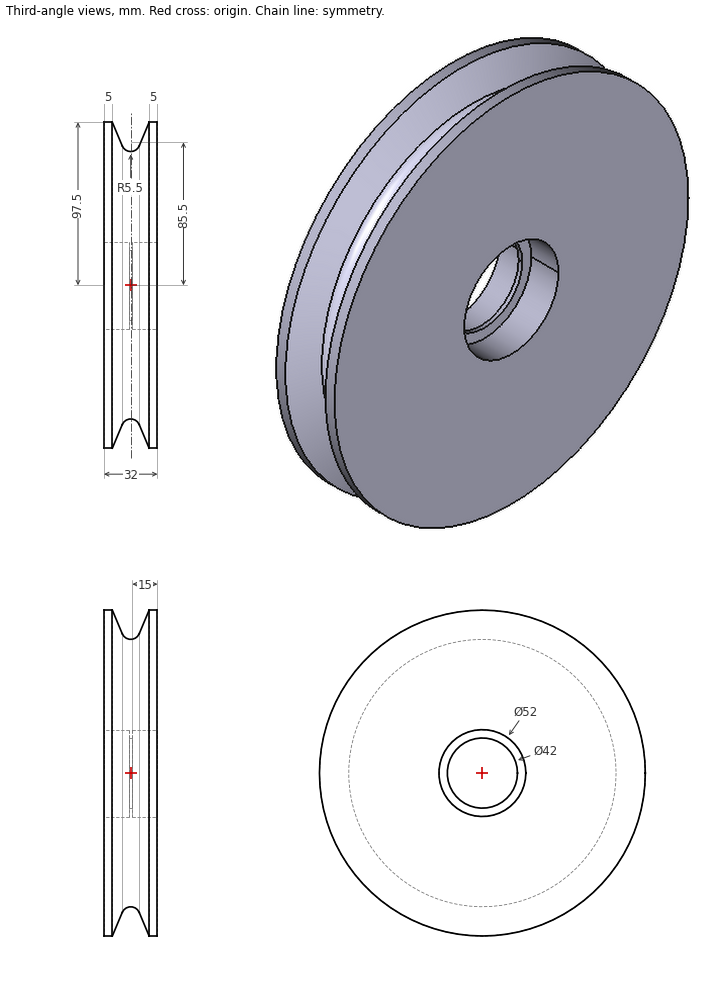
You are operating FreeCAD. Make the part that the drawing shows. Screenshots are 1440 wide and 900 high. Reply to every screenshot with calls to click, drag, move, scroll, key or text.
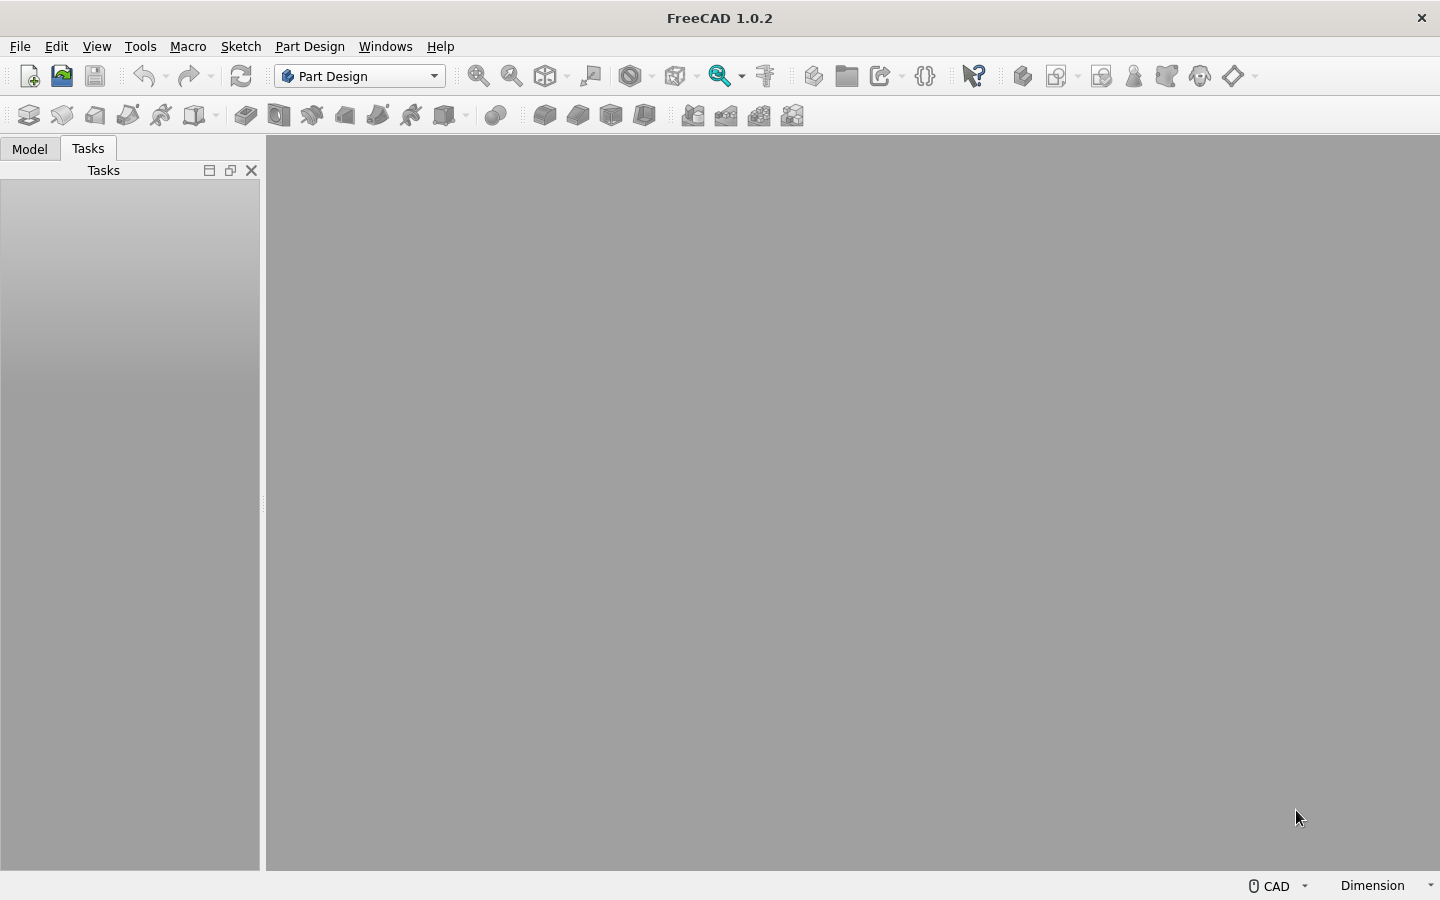
click(29, 76)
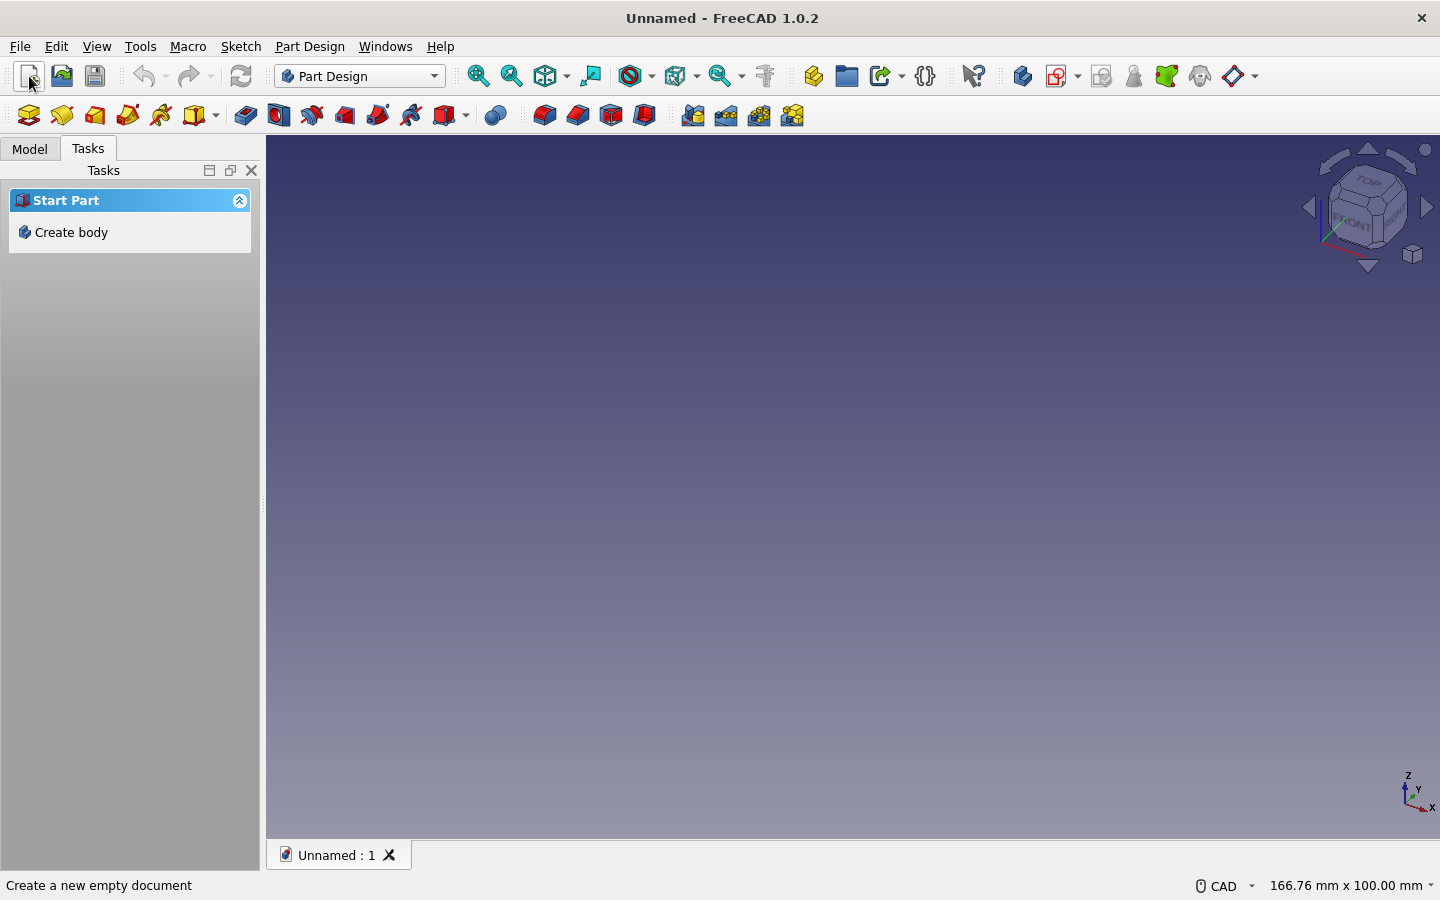
click(1056, 76)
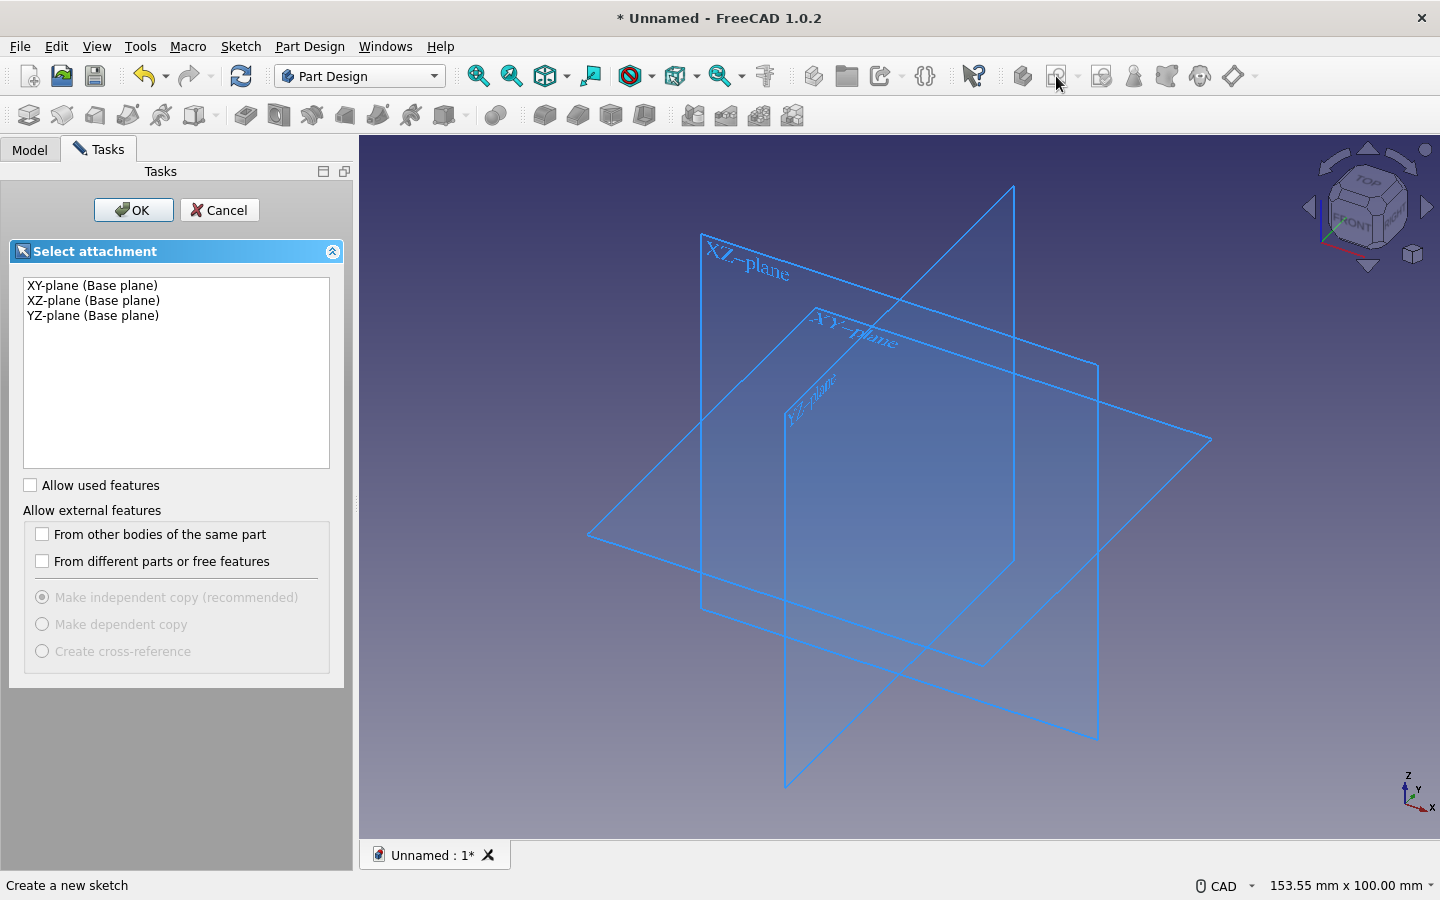
click(84, 286)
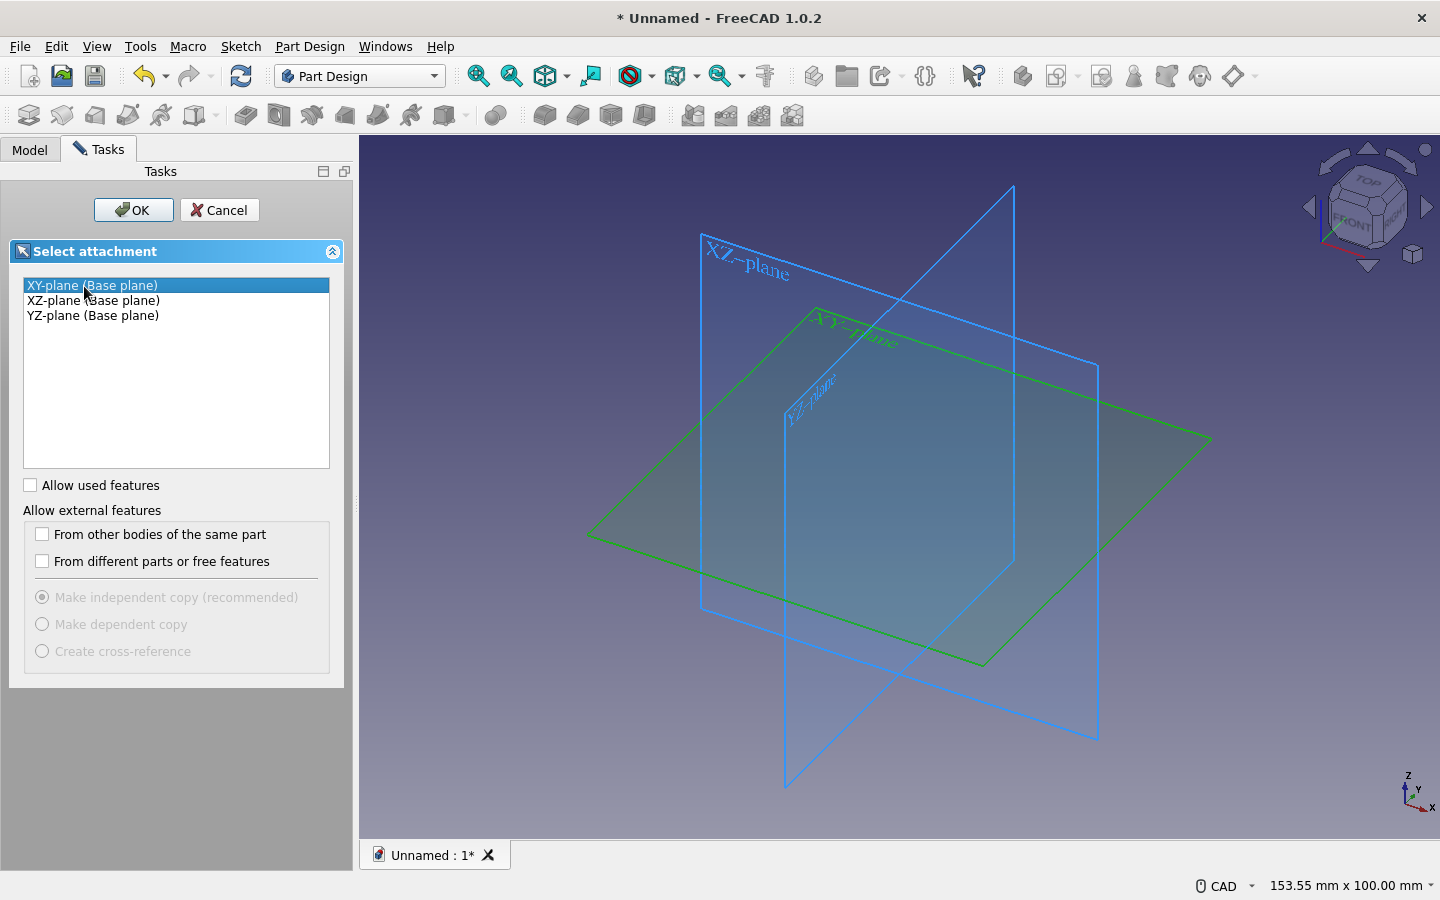
click(134, 210)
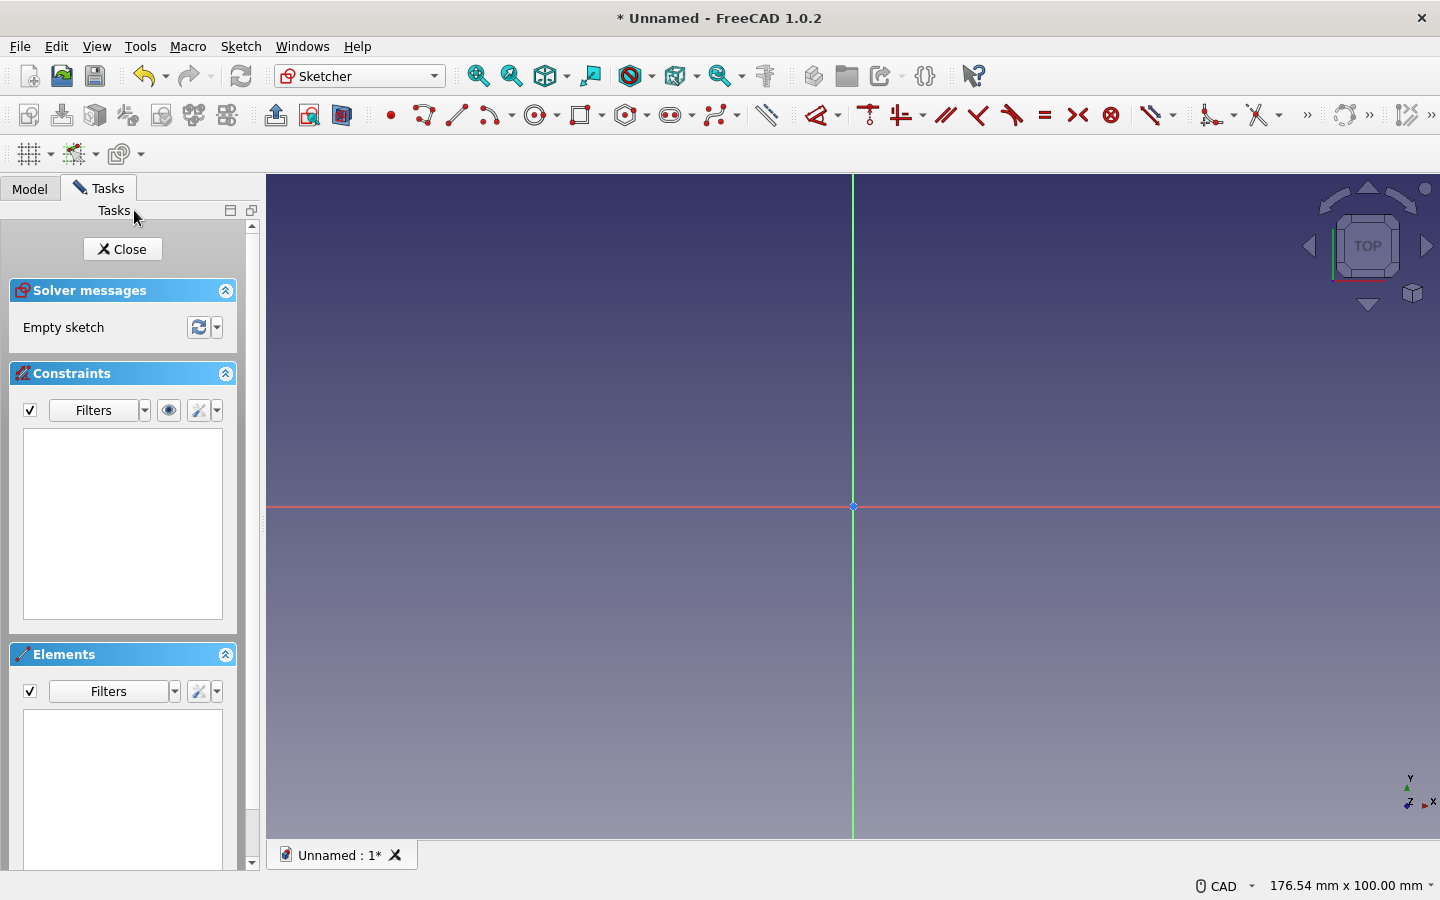
scroll(701, 811, down, 3)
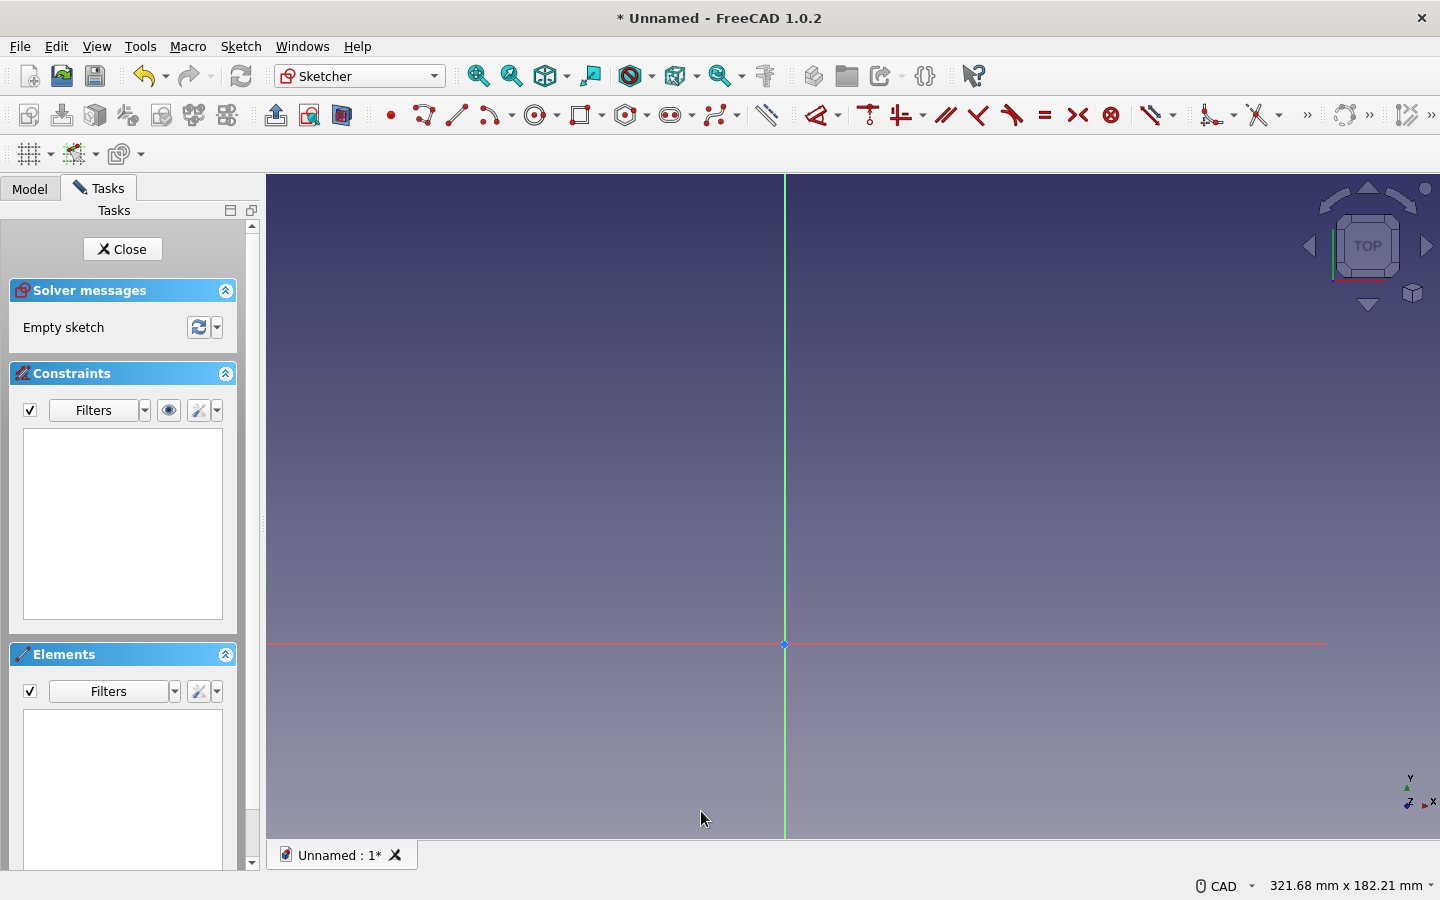
click(424, 116)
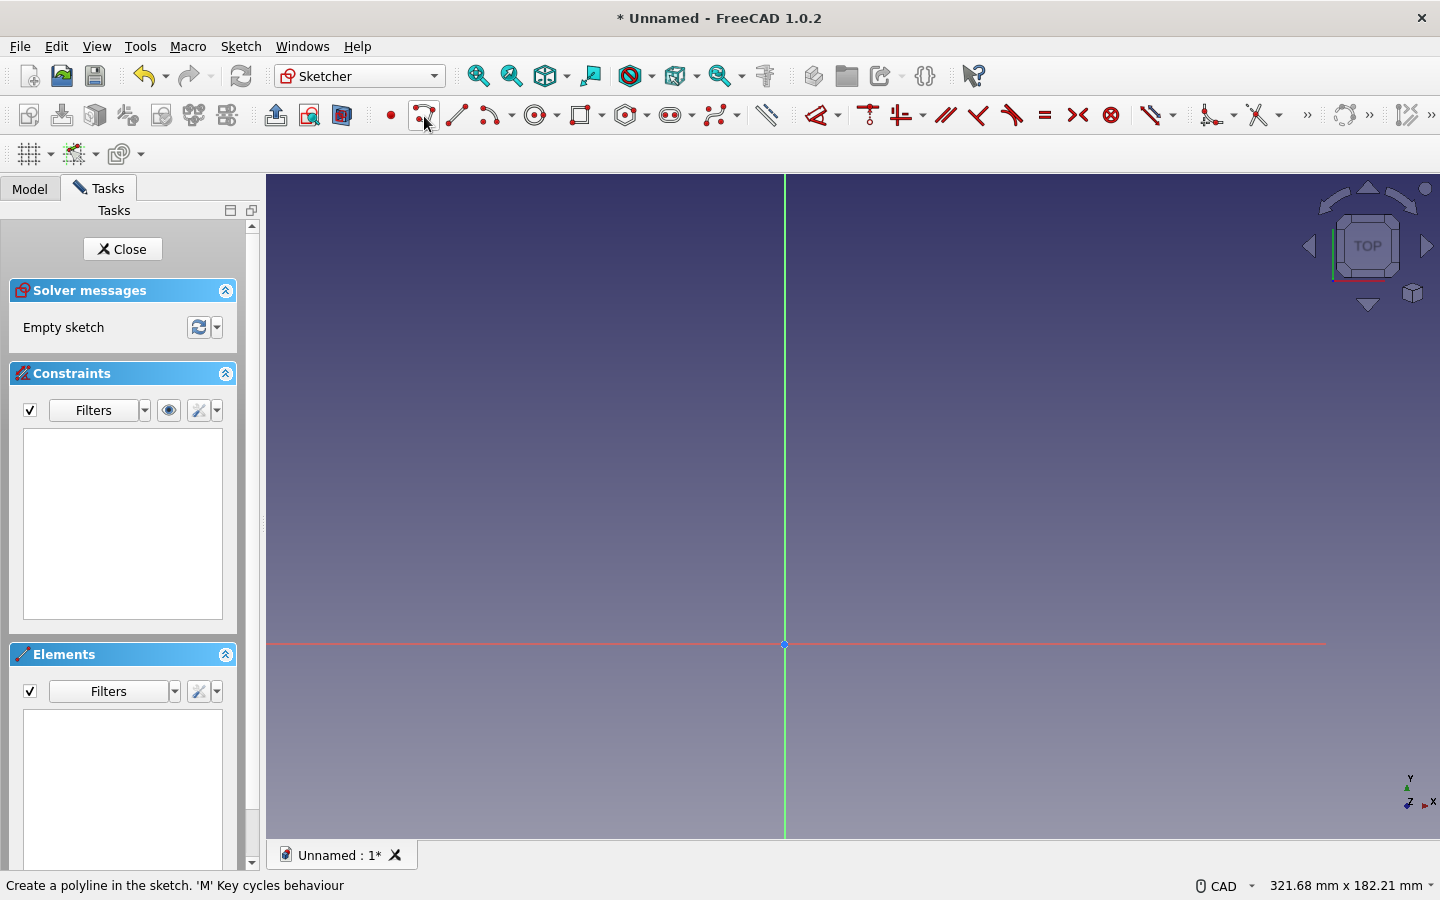
click(766, 340)
click(744, 288)
click(726, 288)
click(726, 644)
click(843, 635)
click(843, 288)
click(825, 288)
click(803, 340)
right_click(803, 340)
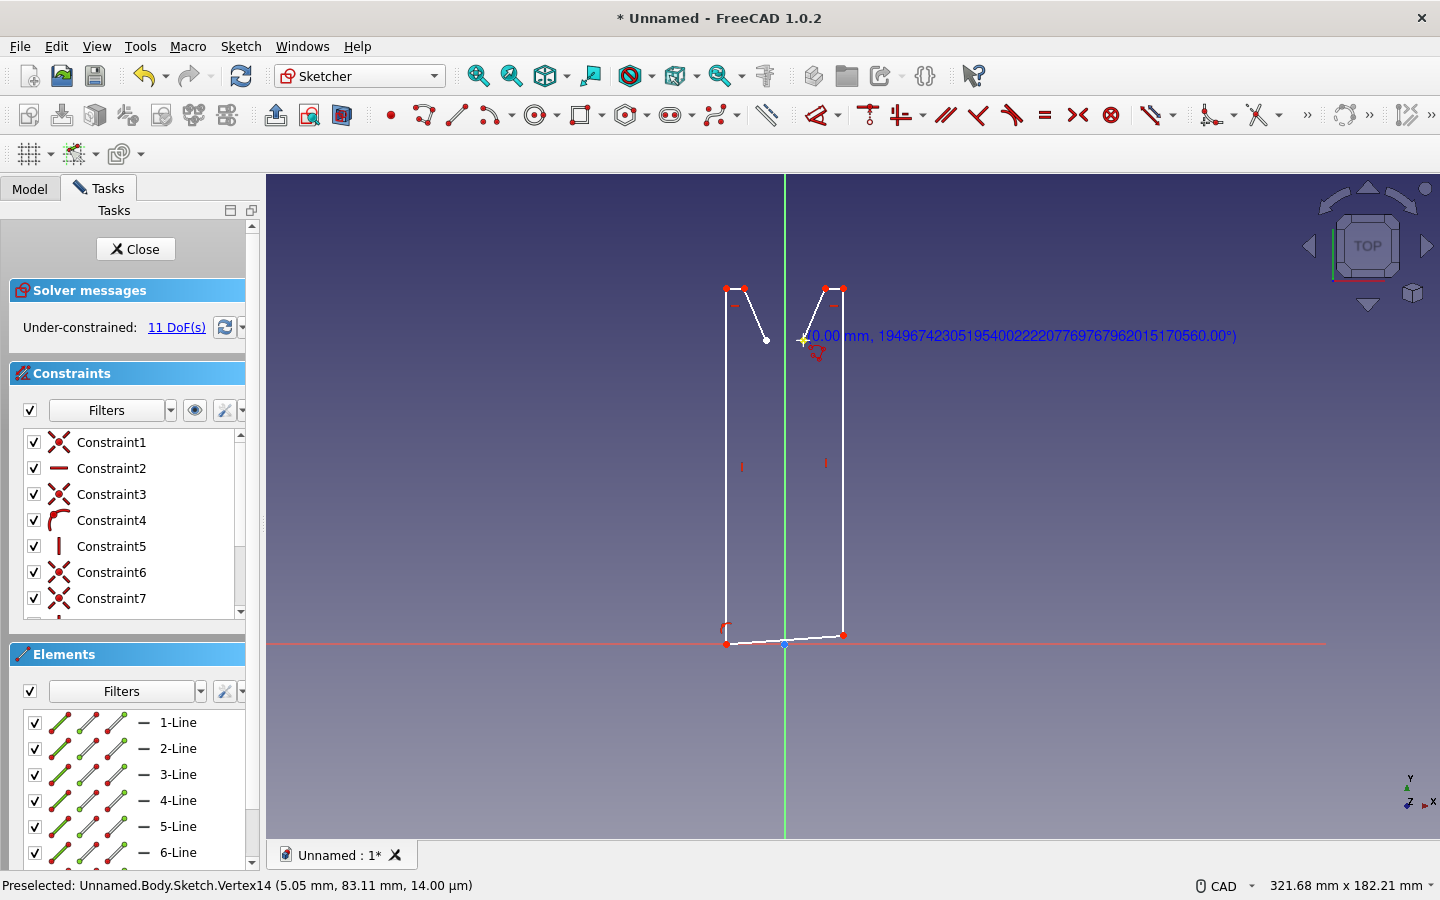
click(512, 116)